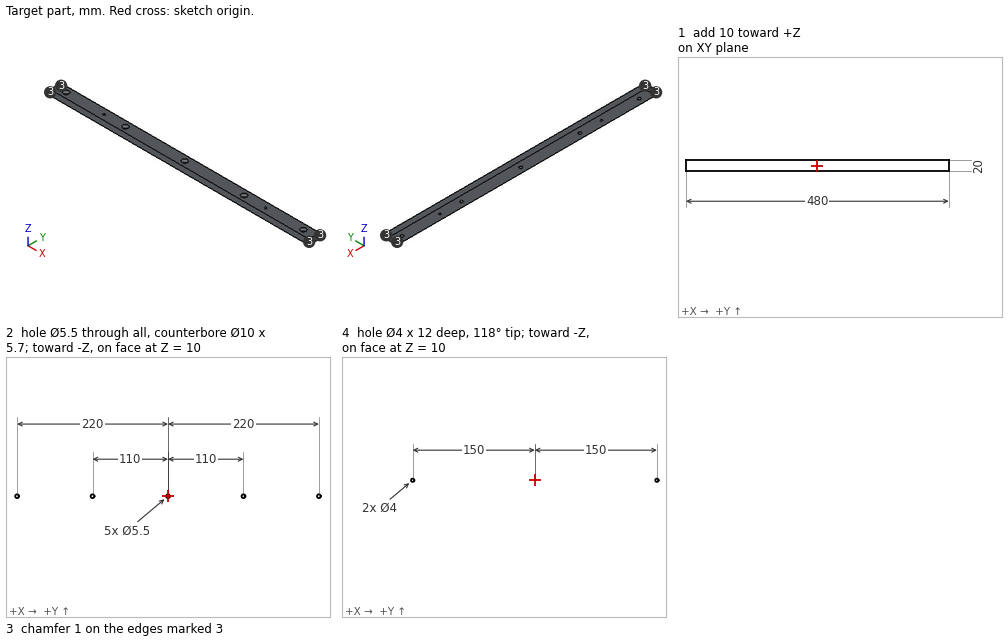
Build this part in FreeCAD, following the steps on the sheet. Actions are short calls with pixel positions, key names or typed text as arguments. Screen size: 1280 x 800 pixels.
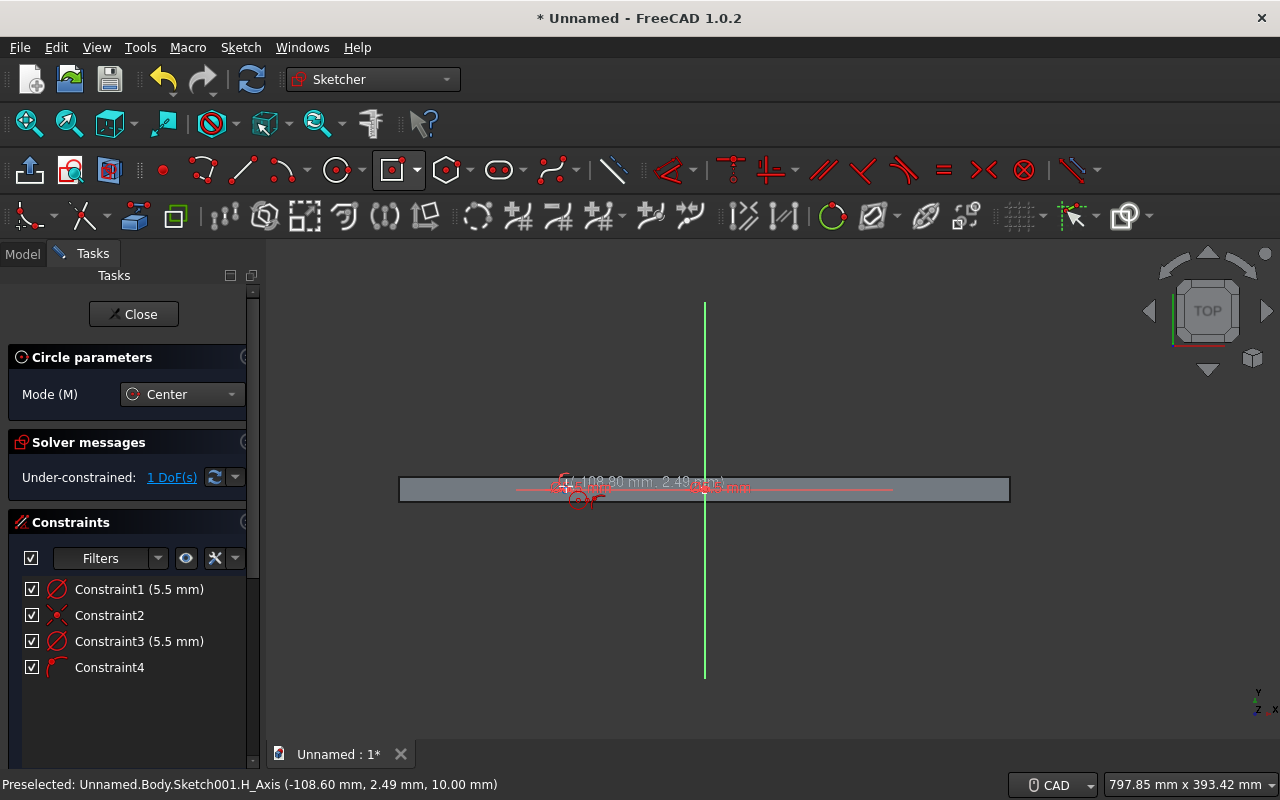
scroll(844, 490, up, 10)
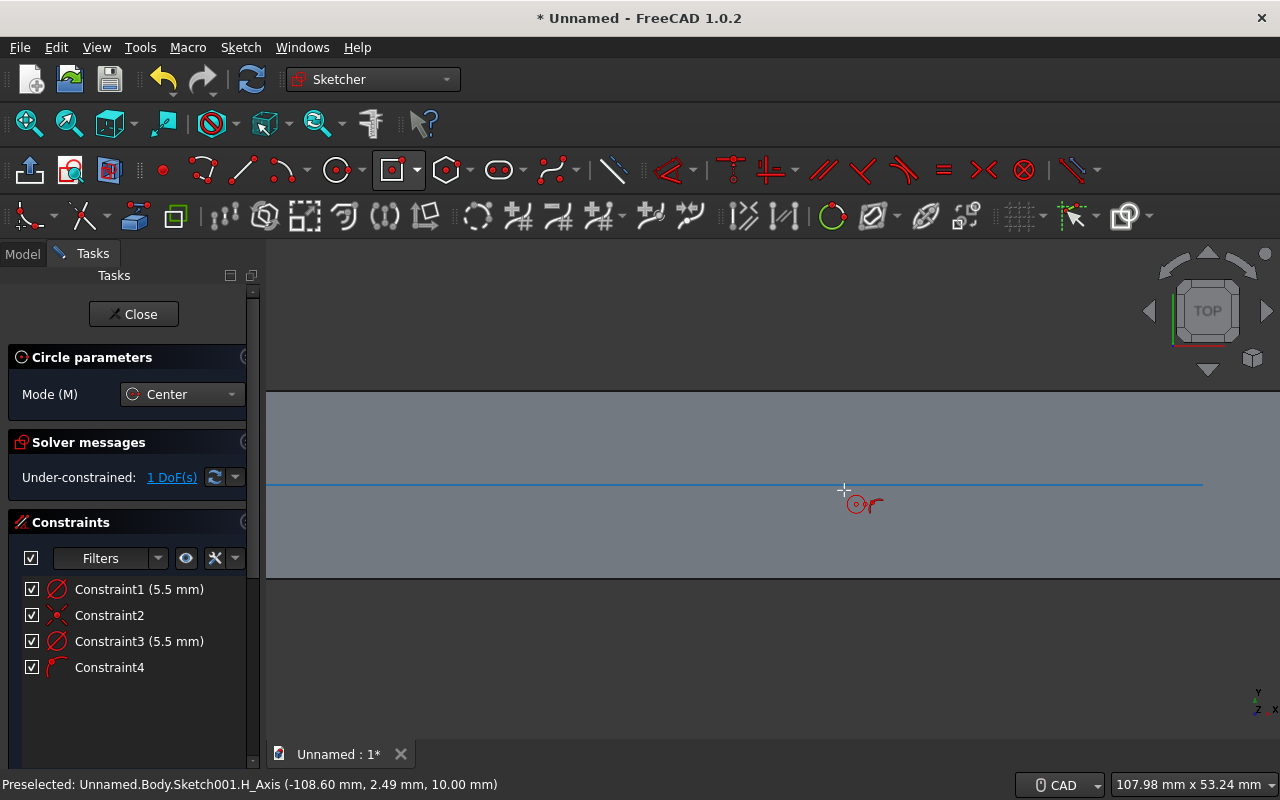
scroll(845, 490, down, 10)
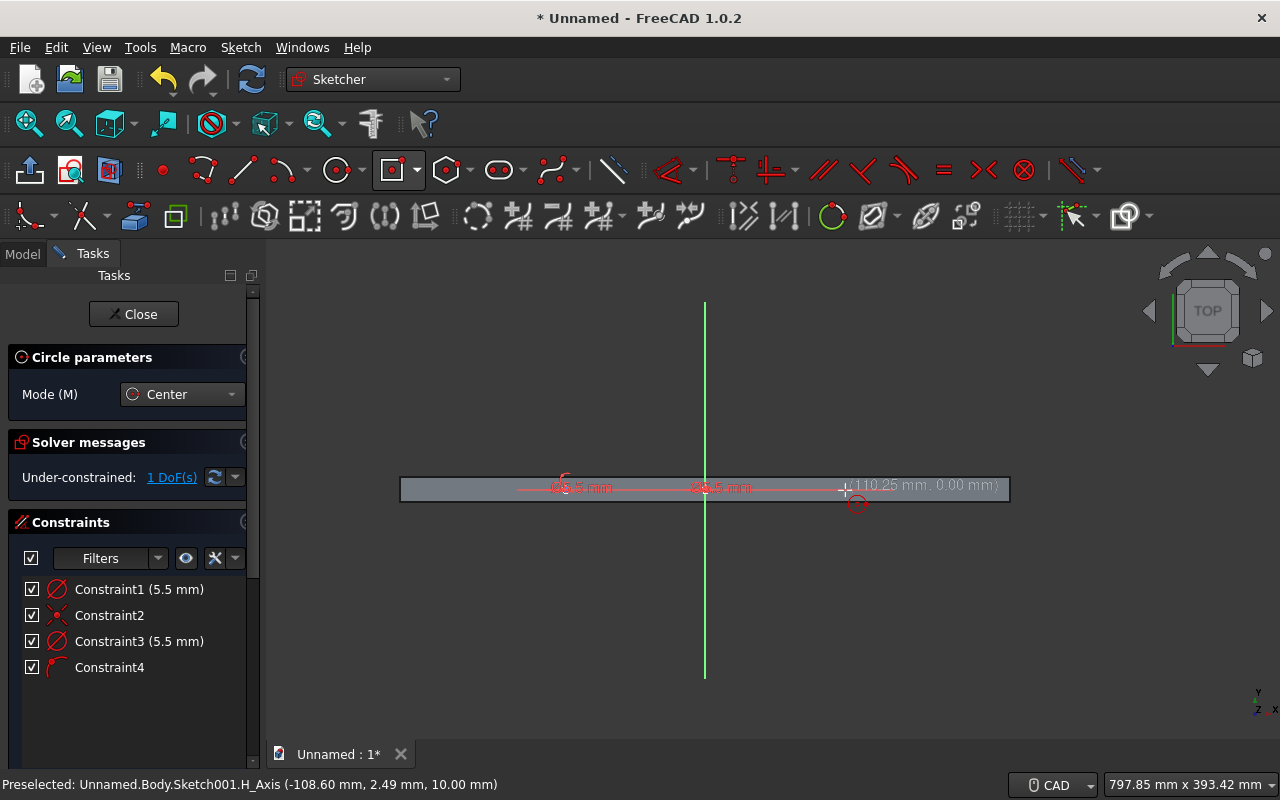
click(845, 490)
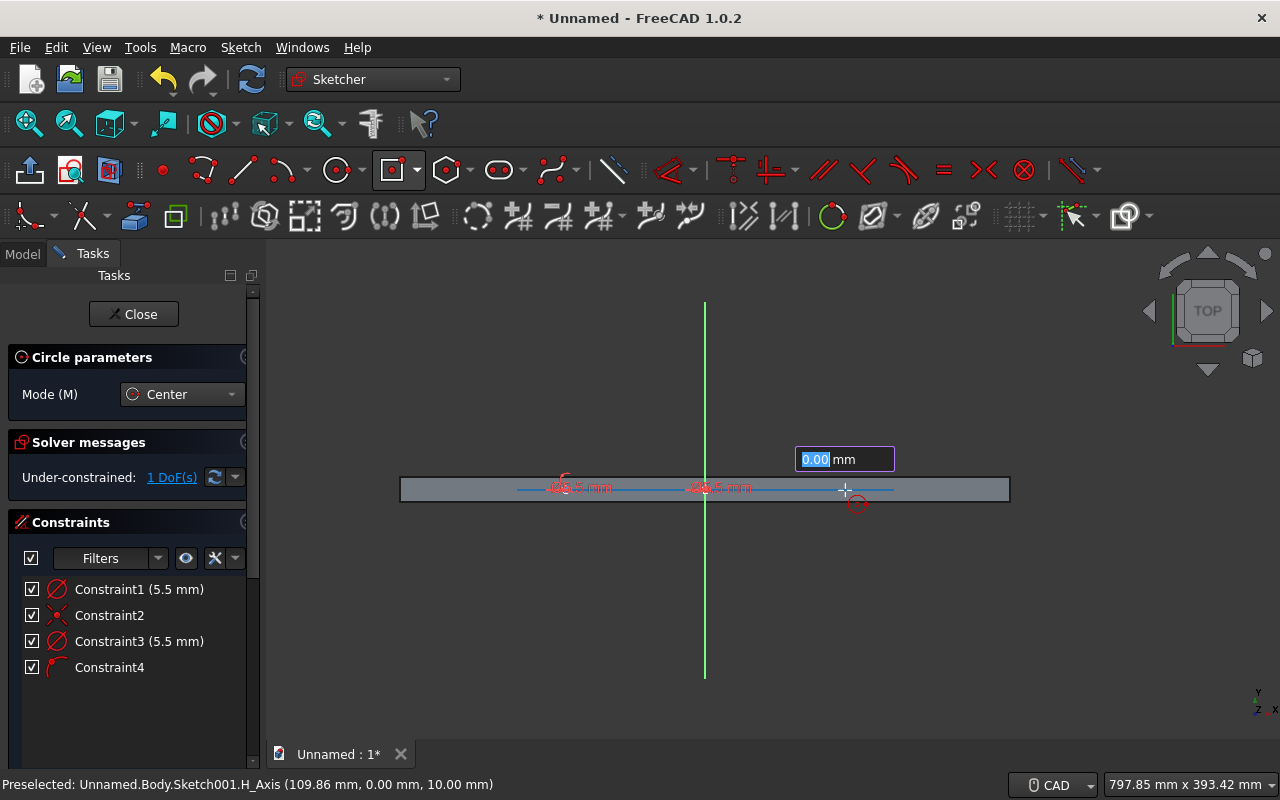
scroll(846, 486, up, 8)
move(846, 486)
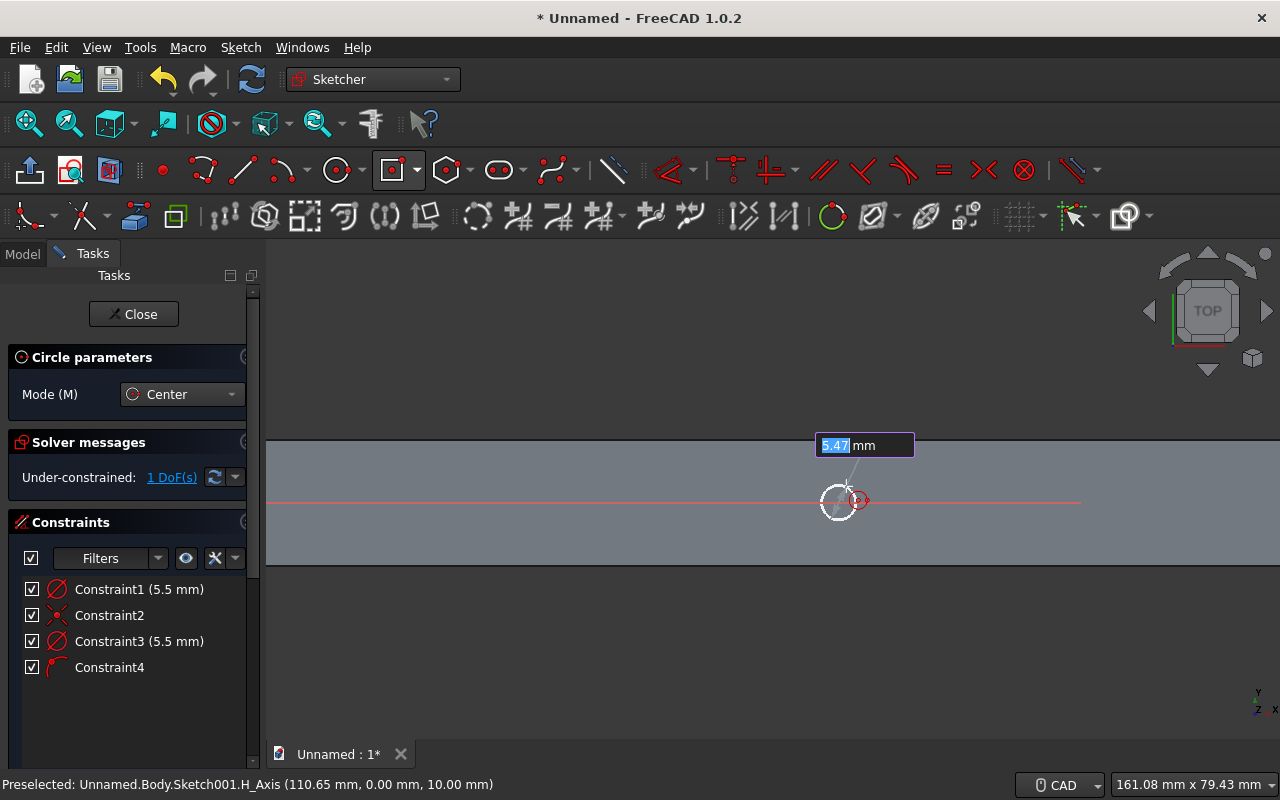
text(5.5)
key(Return)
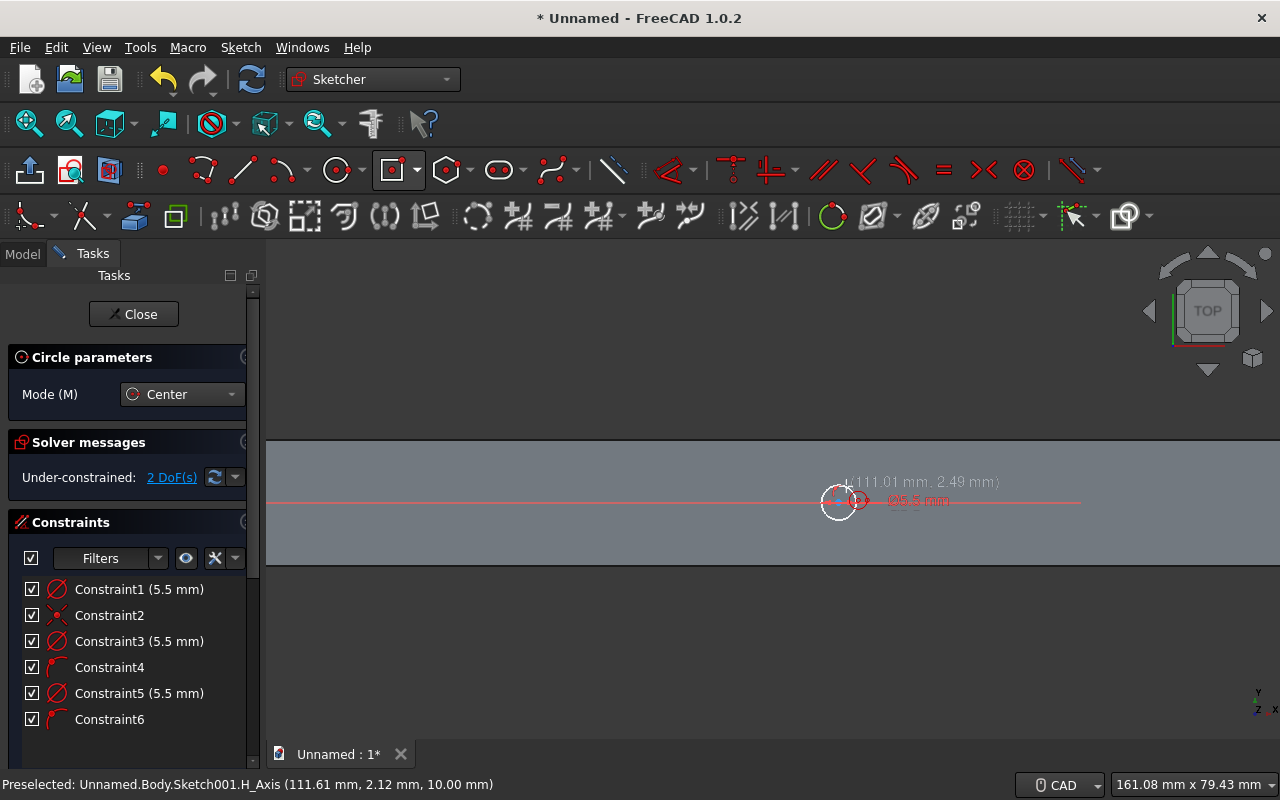
scroll(845, 486, down, 8)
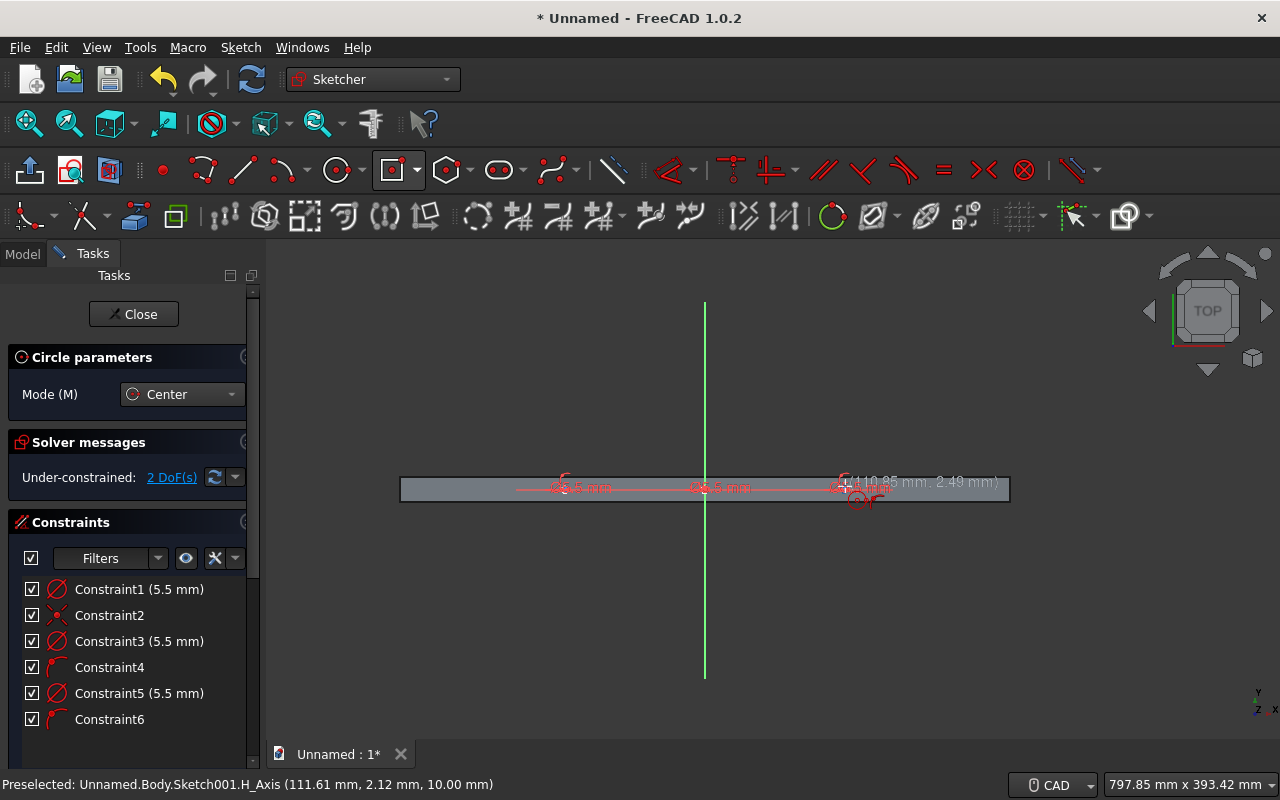
scroll(984, 490, up, 10)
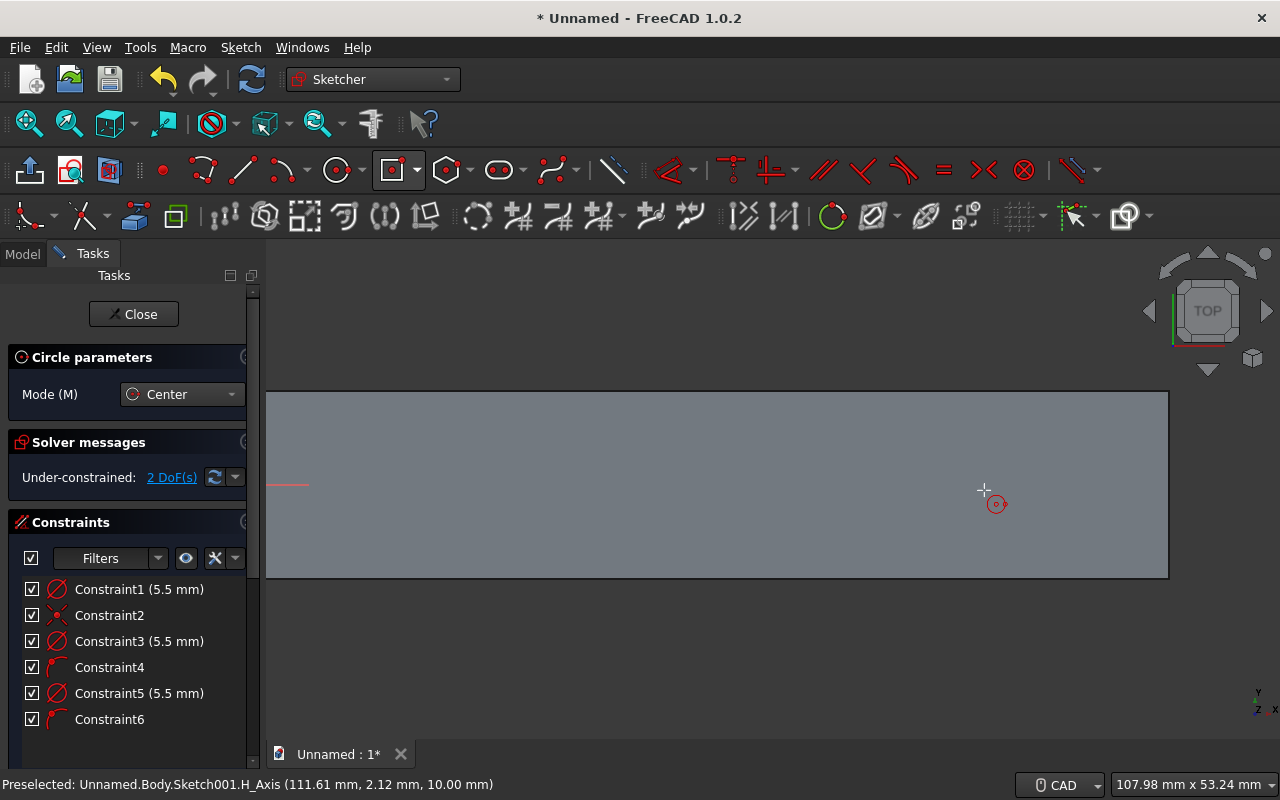
scroll(985, 490, down, 10)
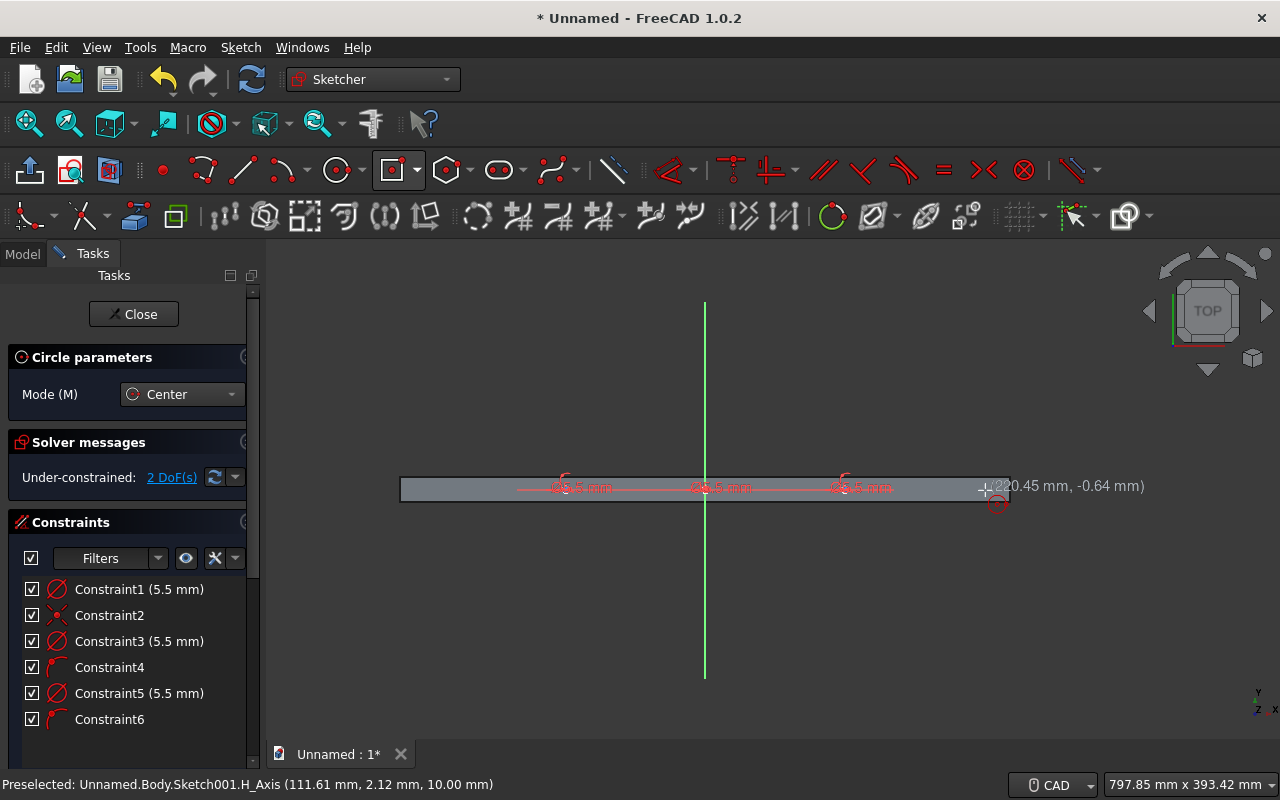
click(985, 490)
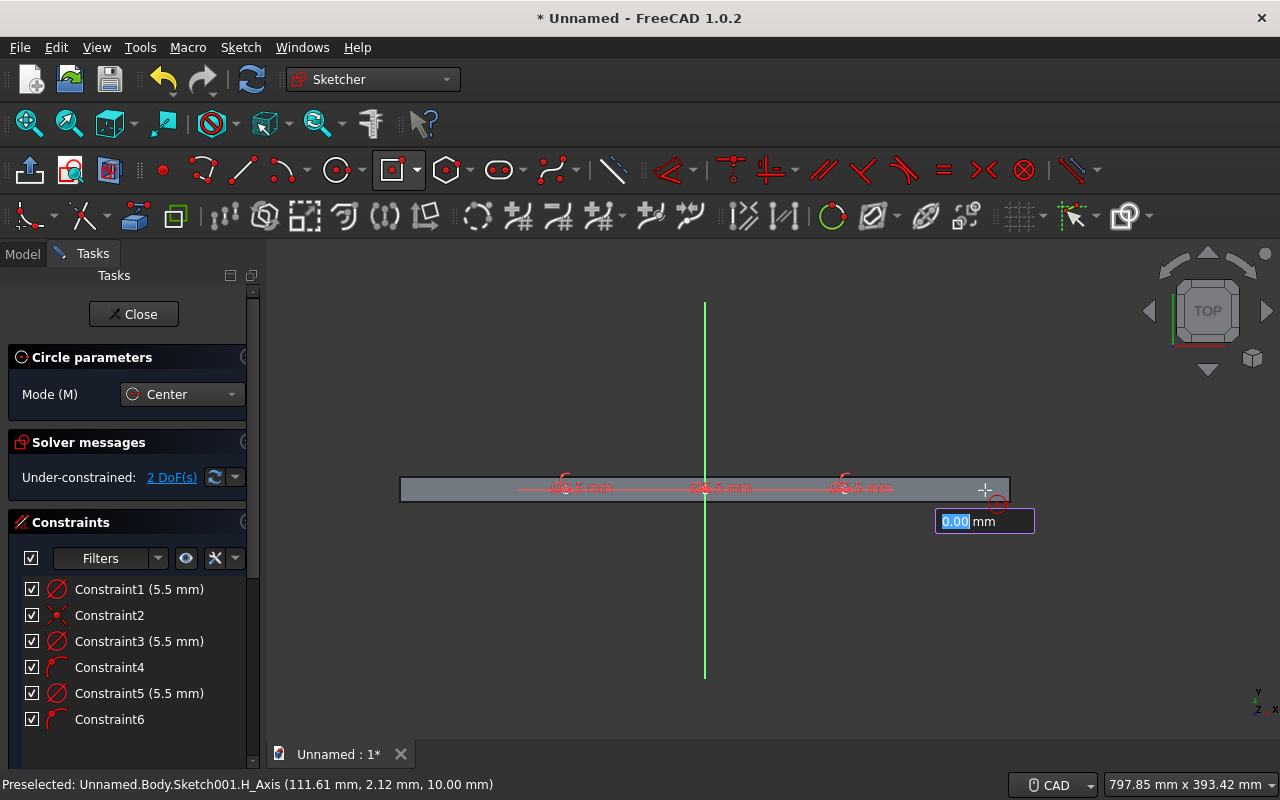
scroll(986, 486, up, 8)
move(984, 486)